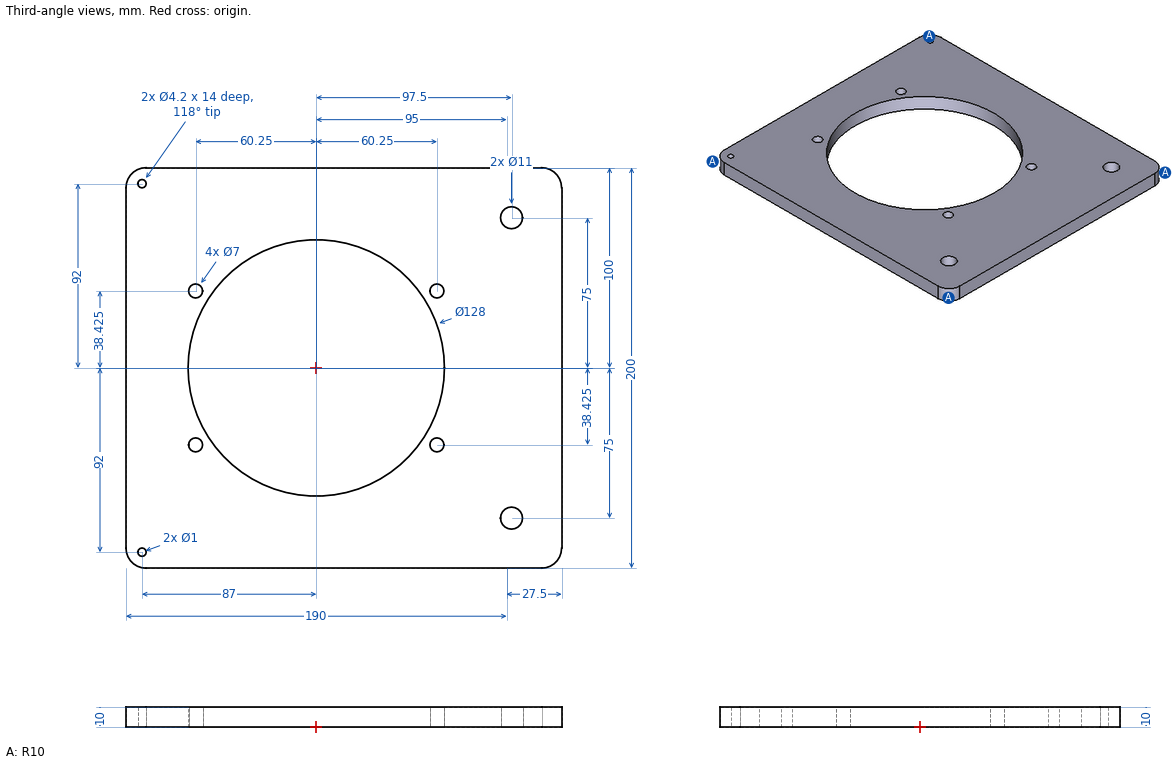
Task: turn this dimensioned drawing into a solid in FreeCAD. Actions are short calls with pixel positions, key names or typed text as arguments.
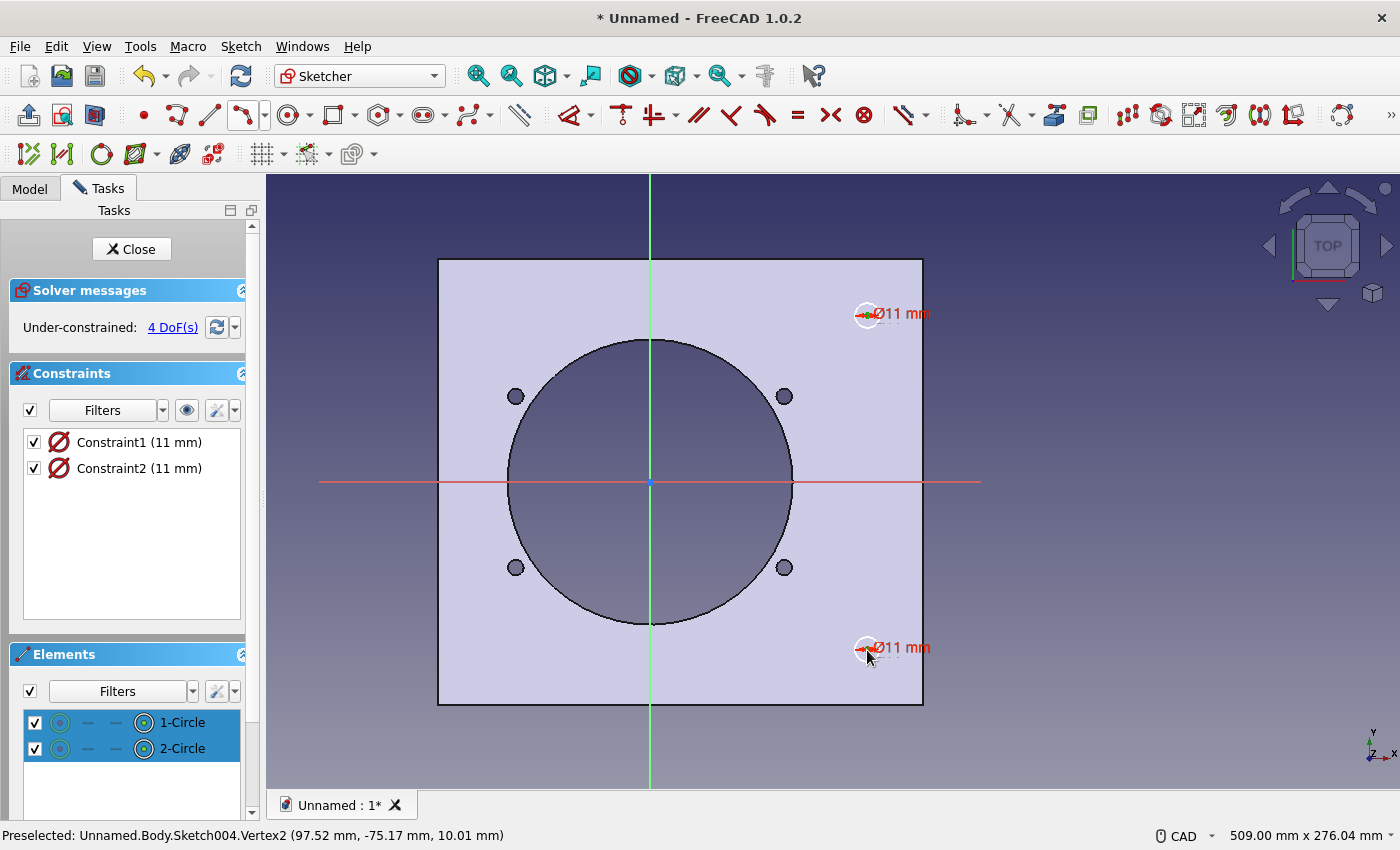
key(v)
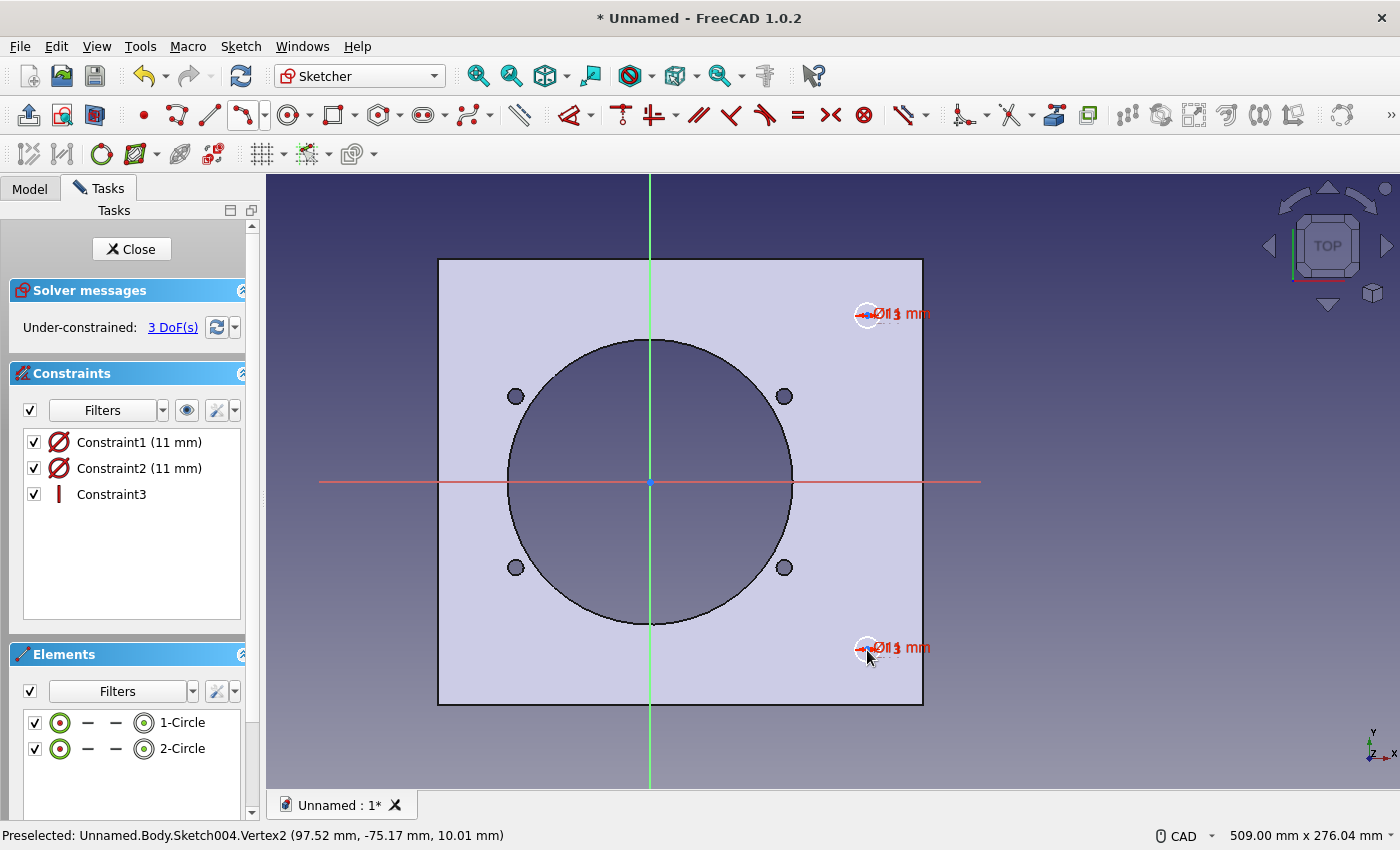
key(d)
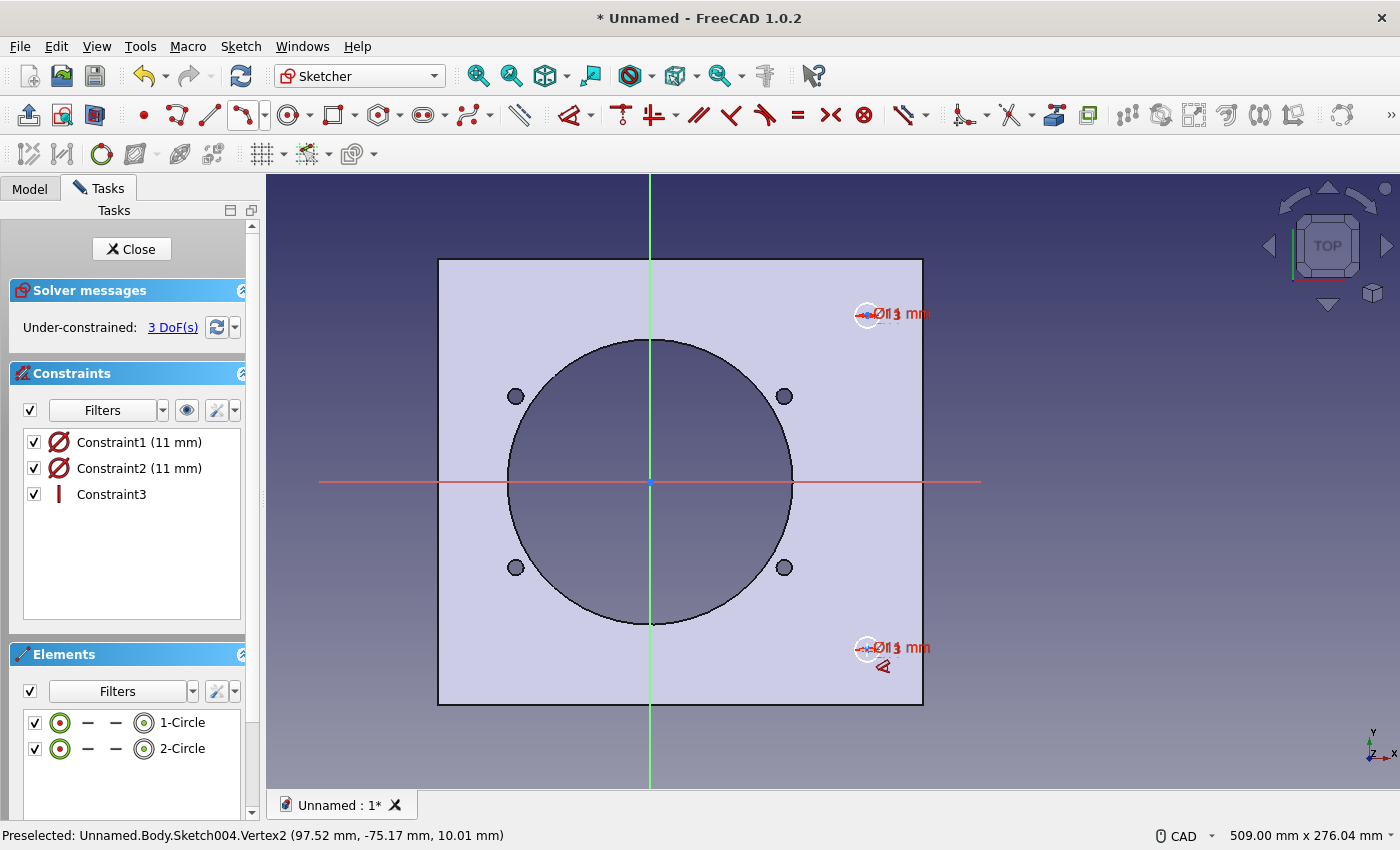
click(867, 316)
click(616, 399)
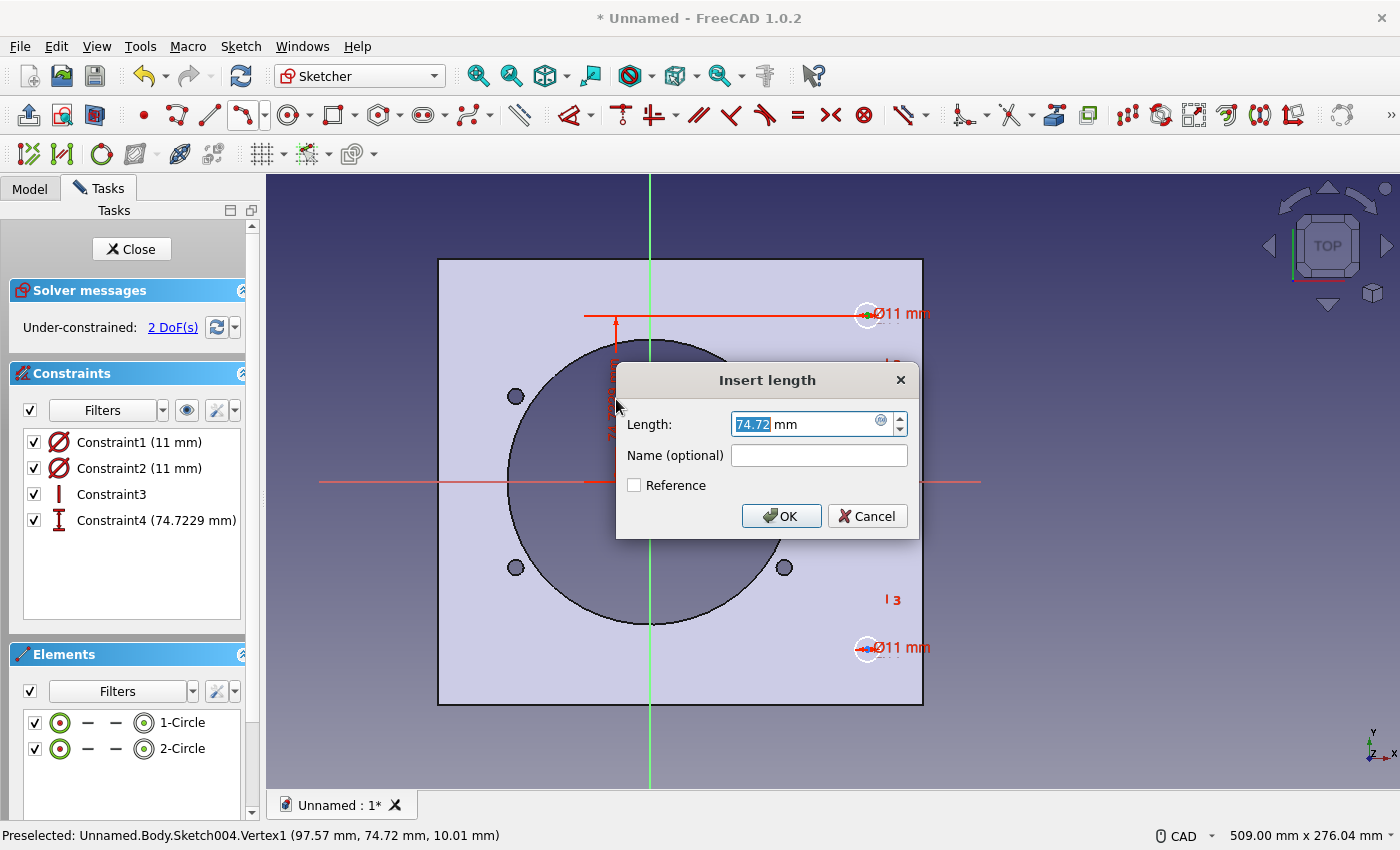
text(75)
key(Return)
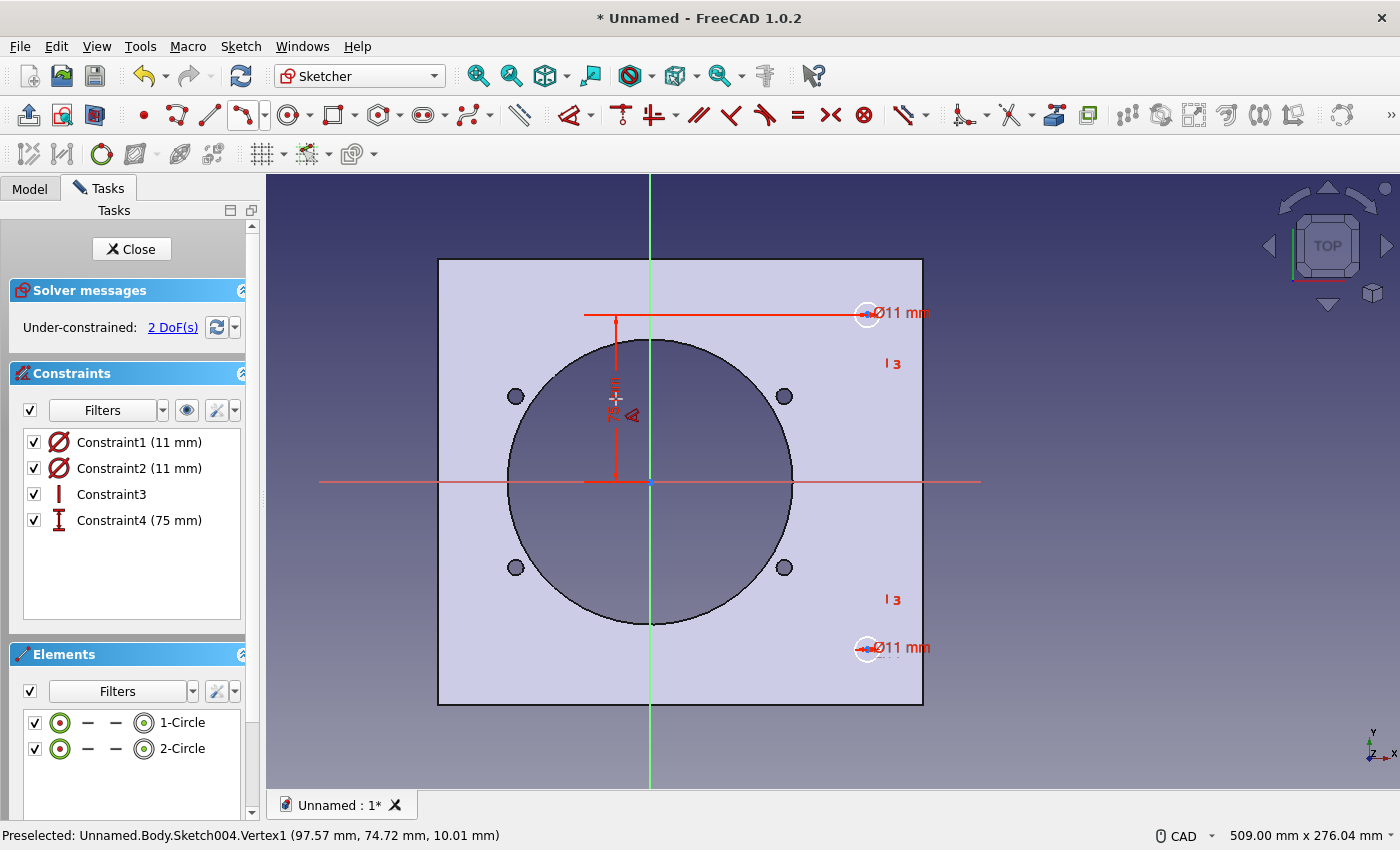
click(867, 650)
click(616, 566)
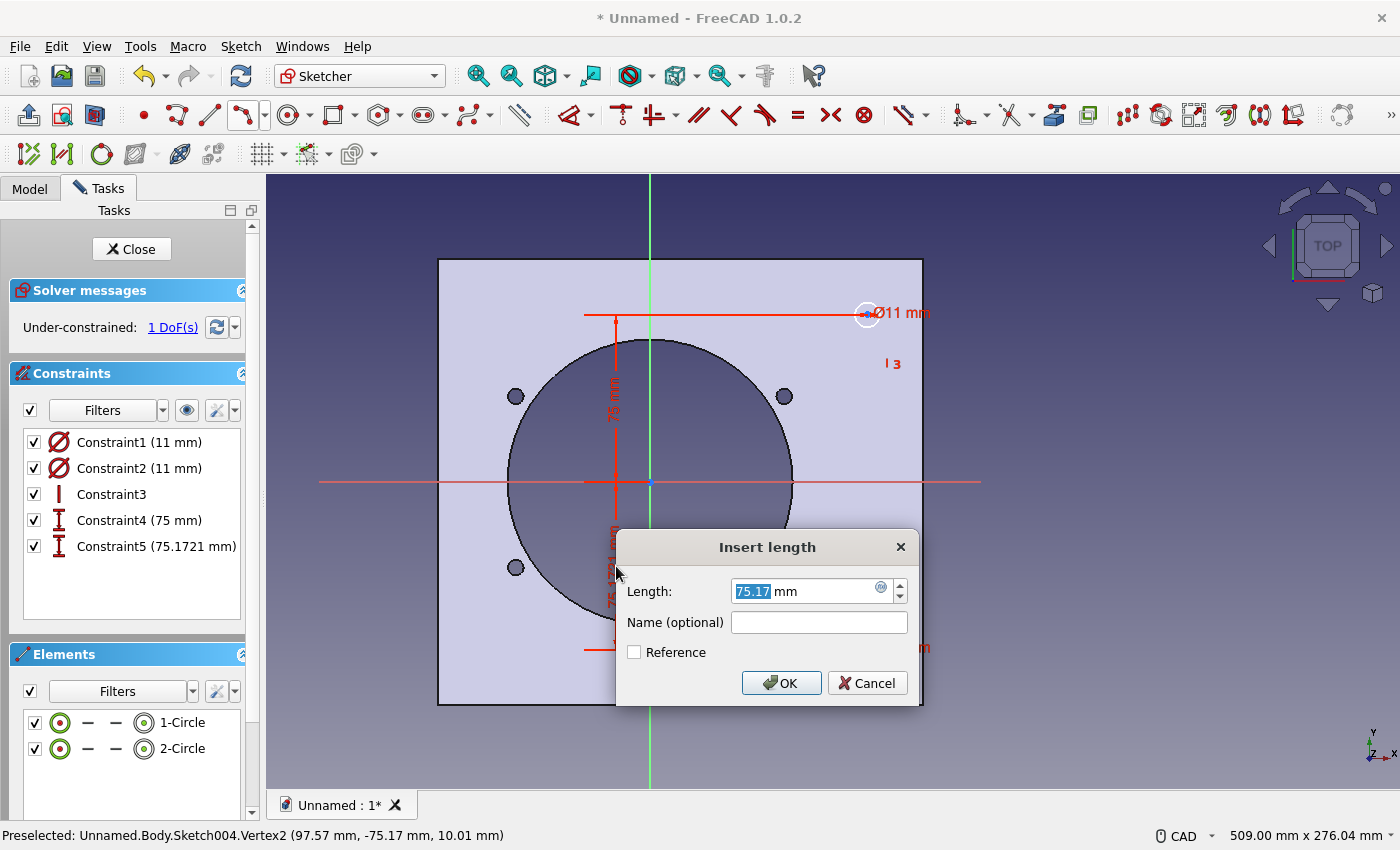
text(75)
key(Return)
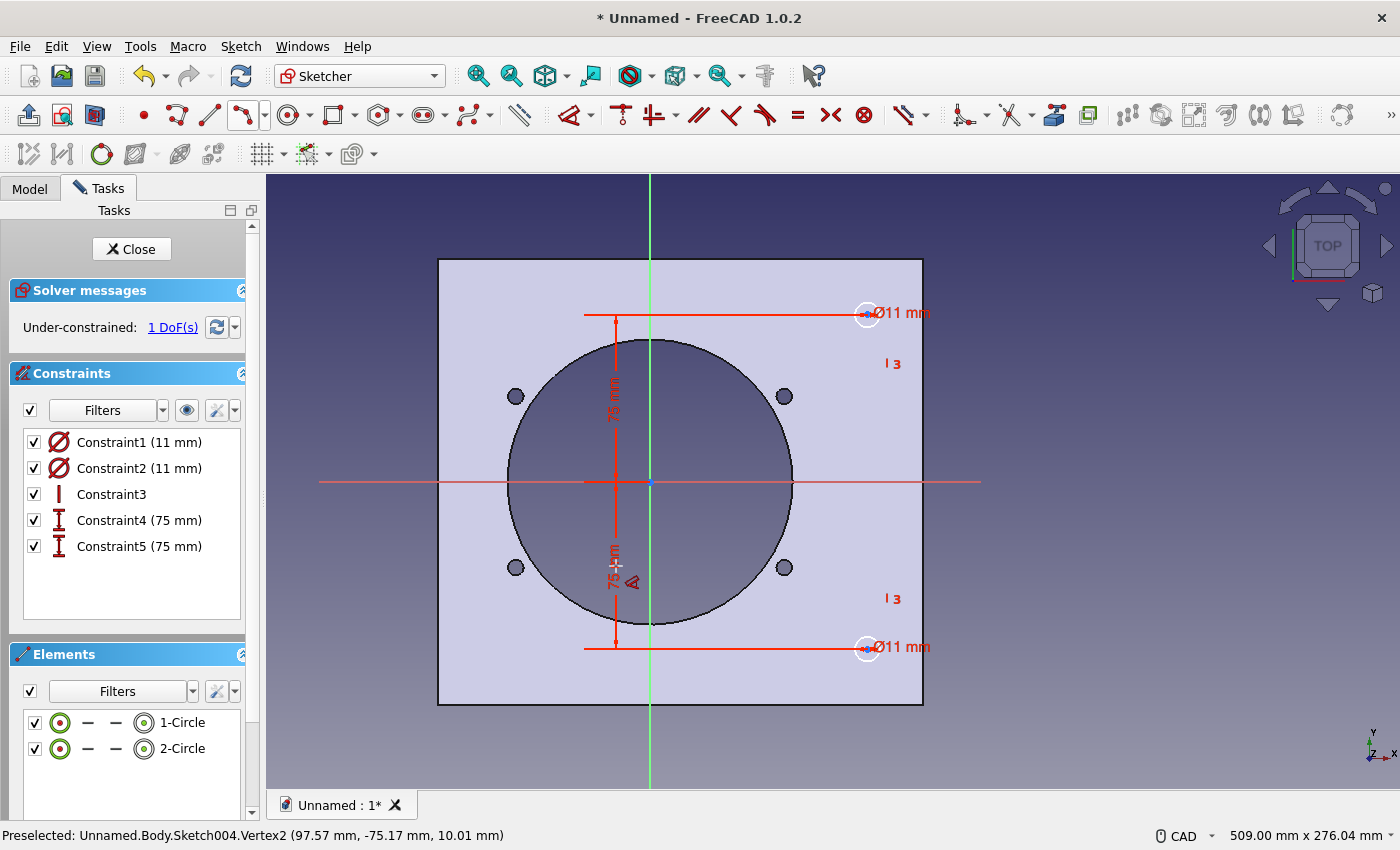
click(867, 315)
click(759, 281)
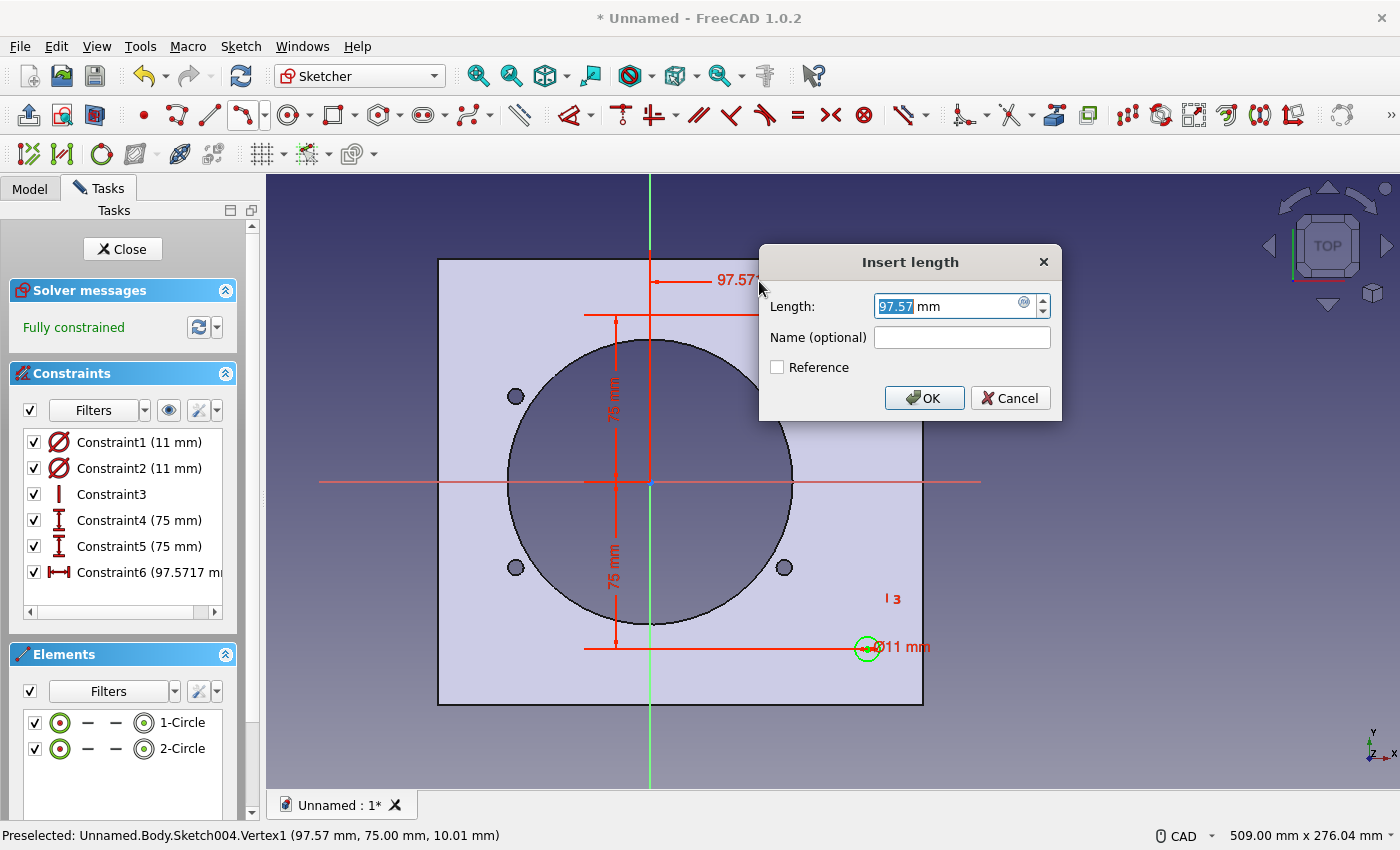
text(97.5)
key(Return)
key(Escape)